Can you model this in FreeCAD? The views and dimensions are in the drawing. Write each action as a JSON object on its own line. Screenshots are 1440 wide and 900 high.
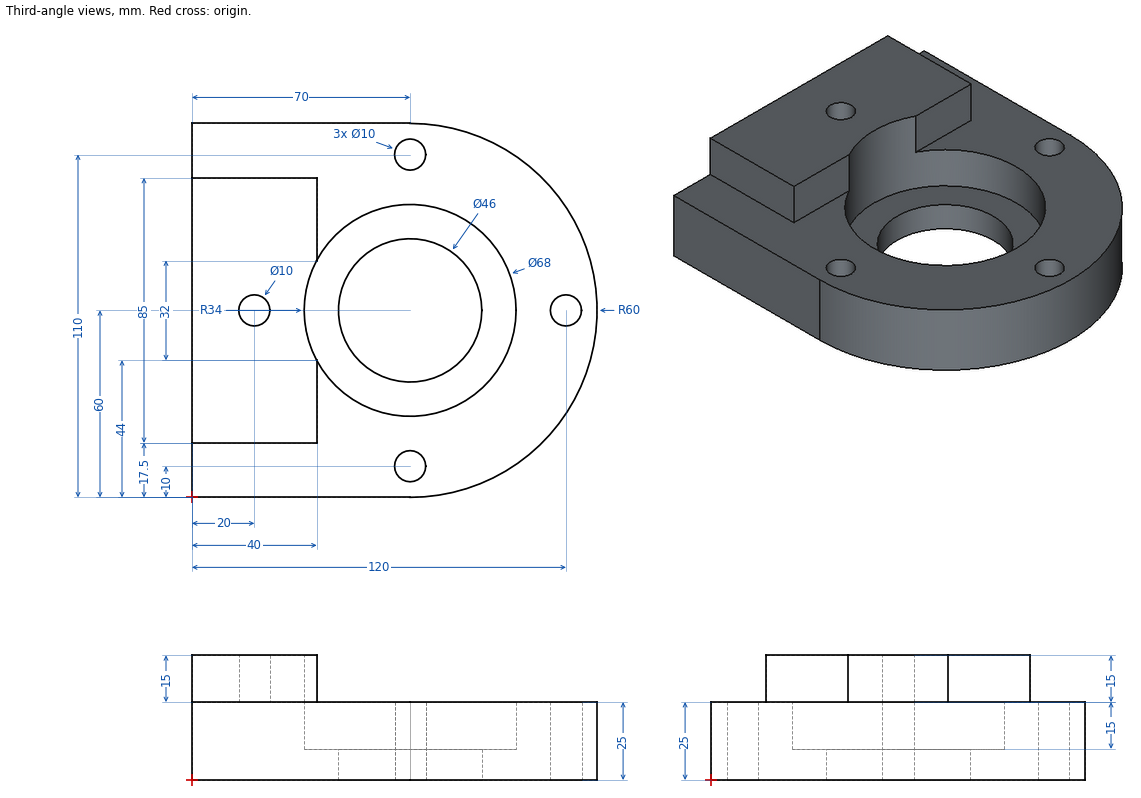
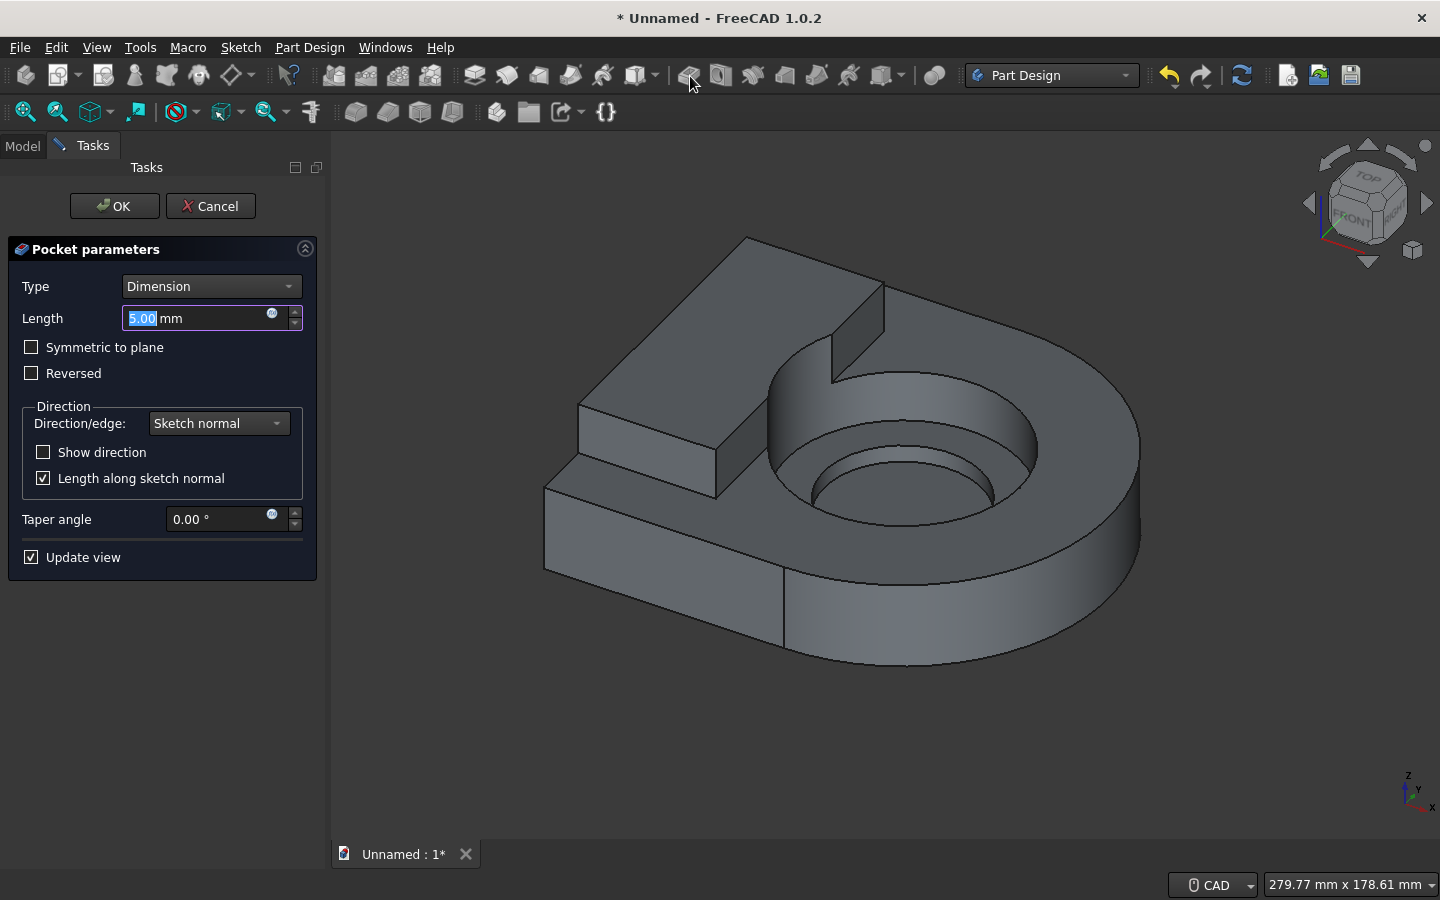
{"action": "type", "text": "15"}
{"action": "key", "text": "Tab"}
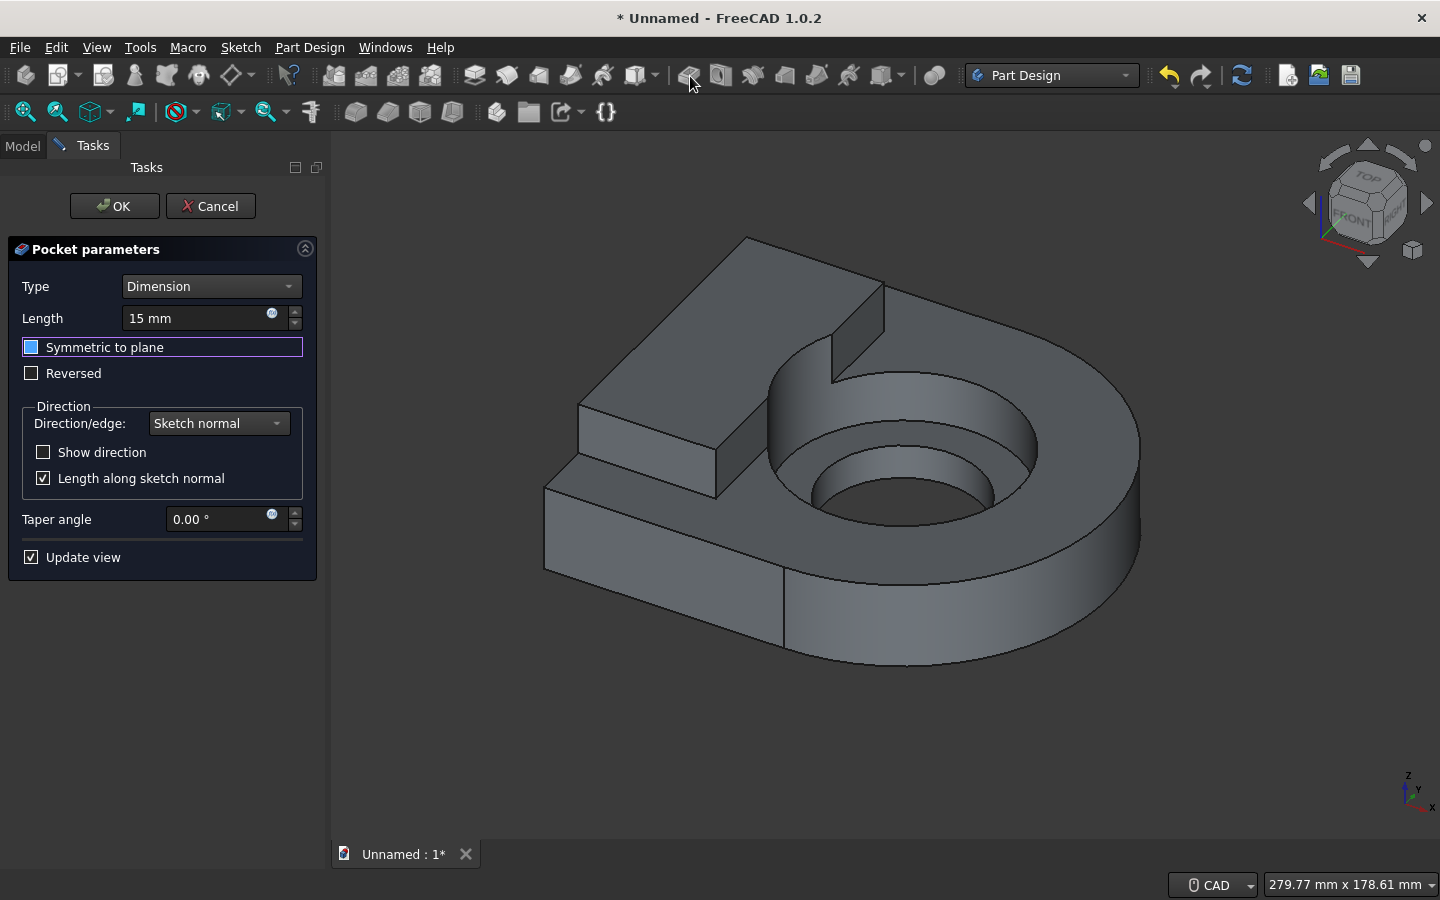
{"action": "left_click", "coordinate": [115, 206]}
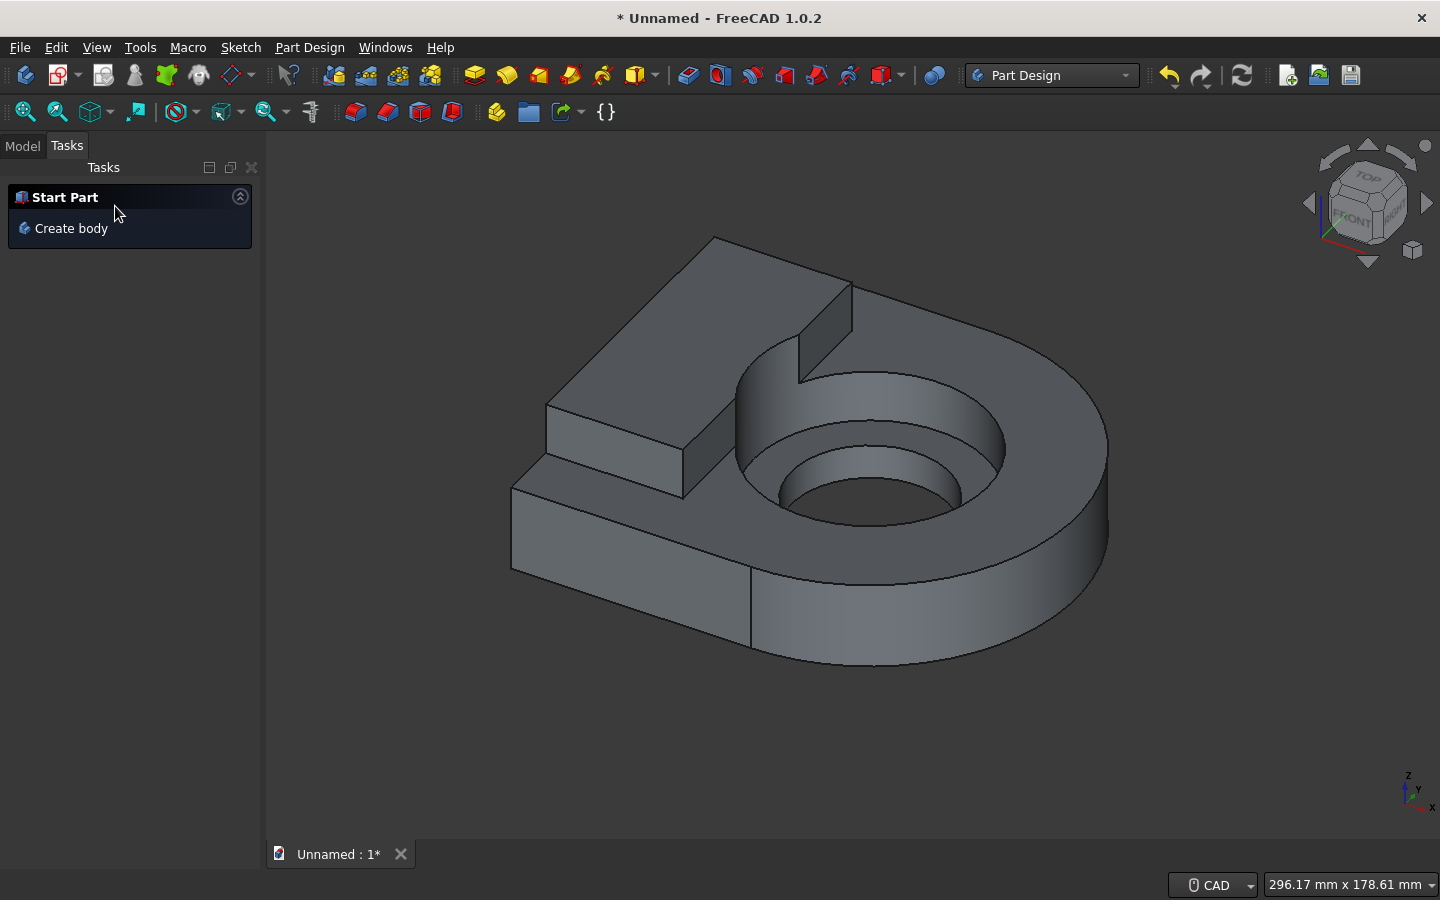
{"action": "left_click", "coordinate": [651, 390]}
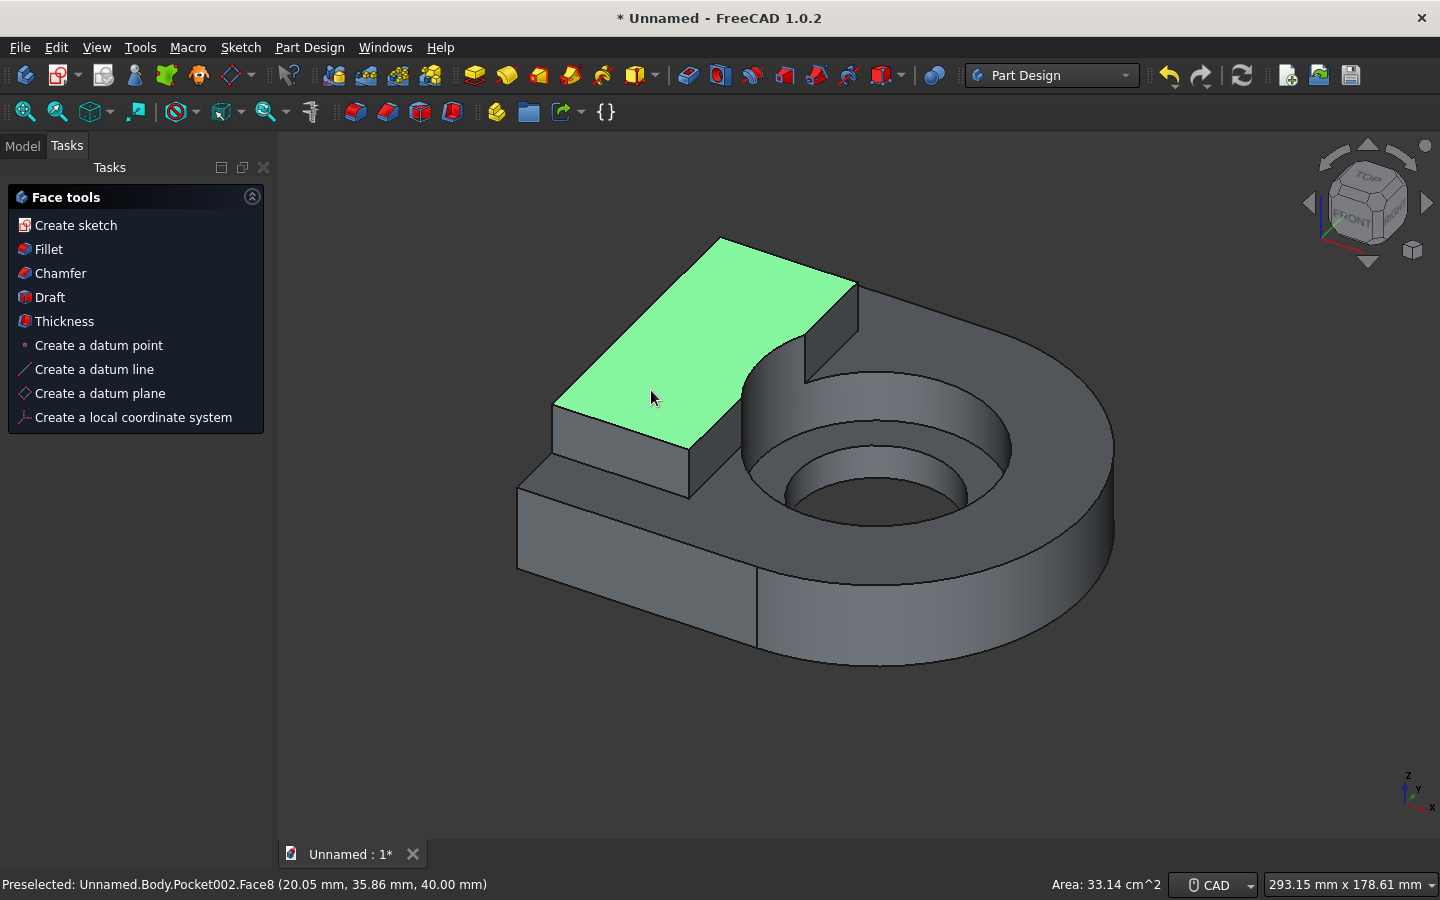
{"action": "left_click", "coordinate": [58, 76]}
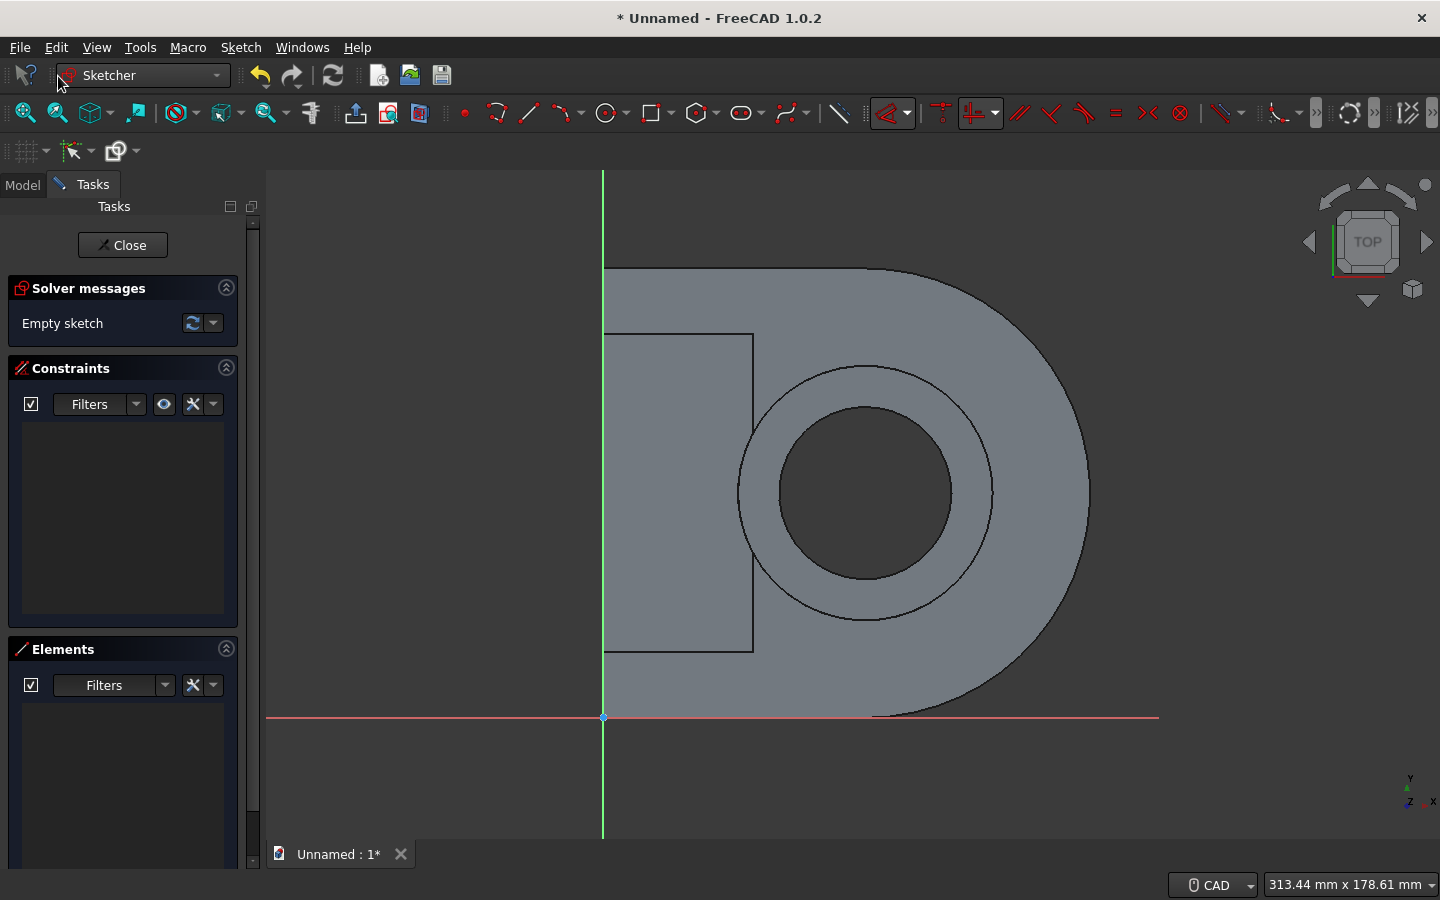
{"action": "scroll", "coordinate": [667, 492], "scroll_direction": "up", "scroll_amount": 12}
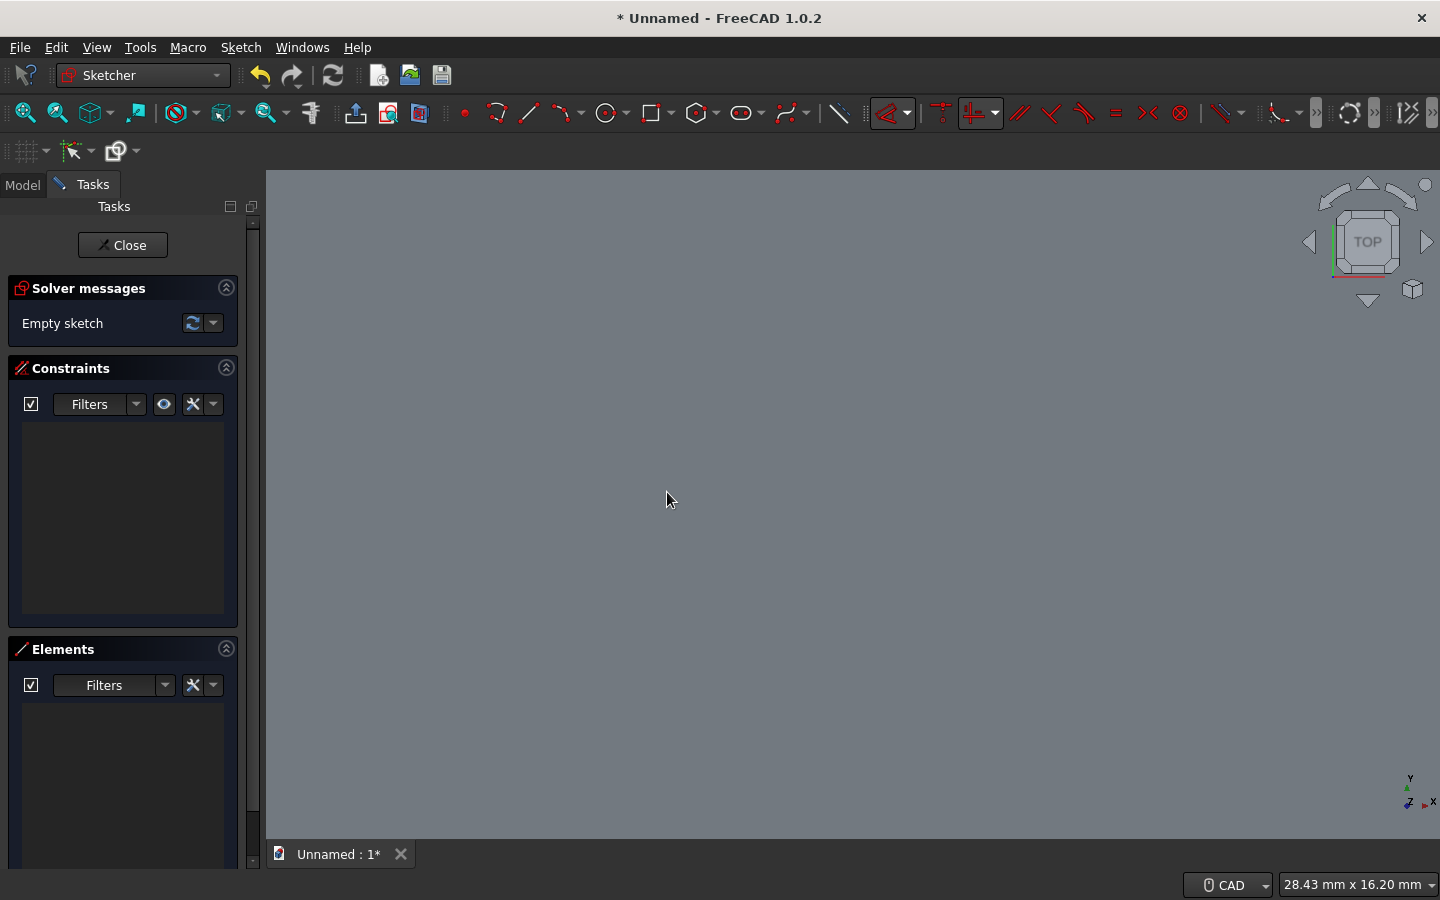
{"action": "left_click", "coordinate": [606, 114]}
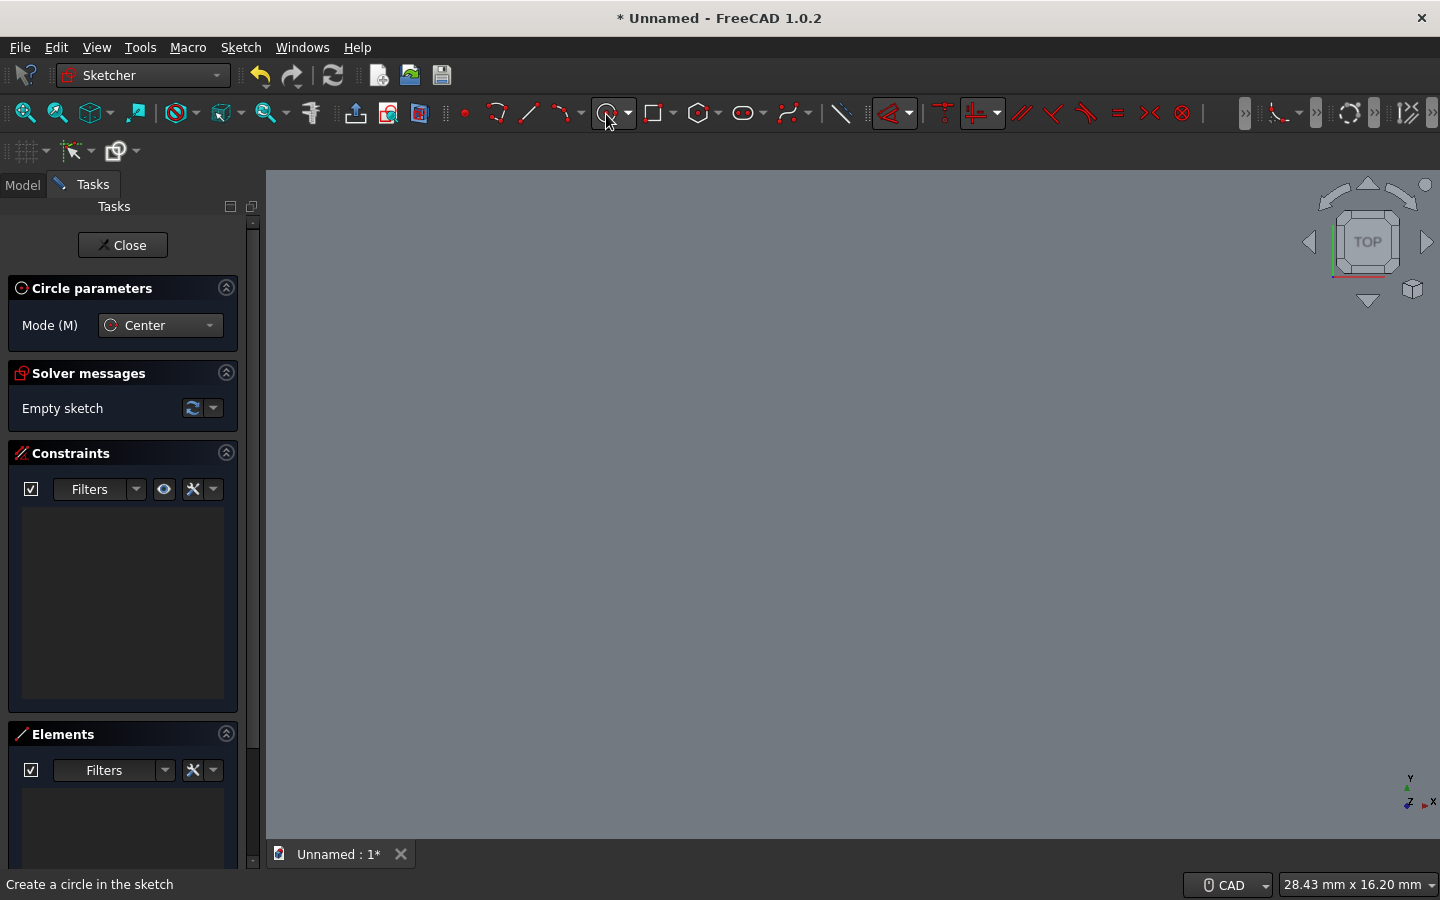
{"action": "left_click", "coordinate": [785, 500]}
{"action": "left_click", "coordinate": [931, 354]}
{"action": "key", "text": "Escape"}